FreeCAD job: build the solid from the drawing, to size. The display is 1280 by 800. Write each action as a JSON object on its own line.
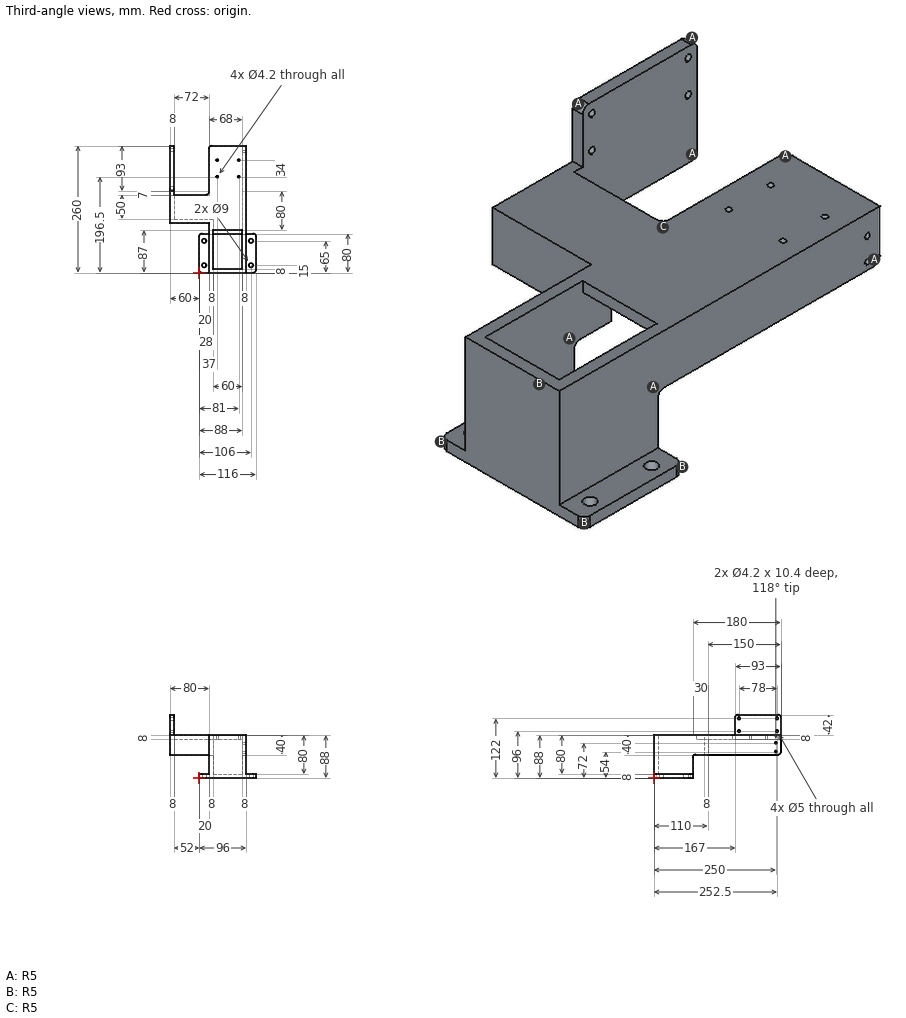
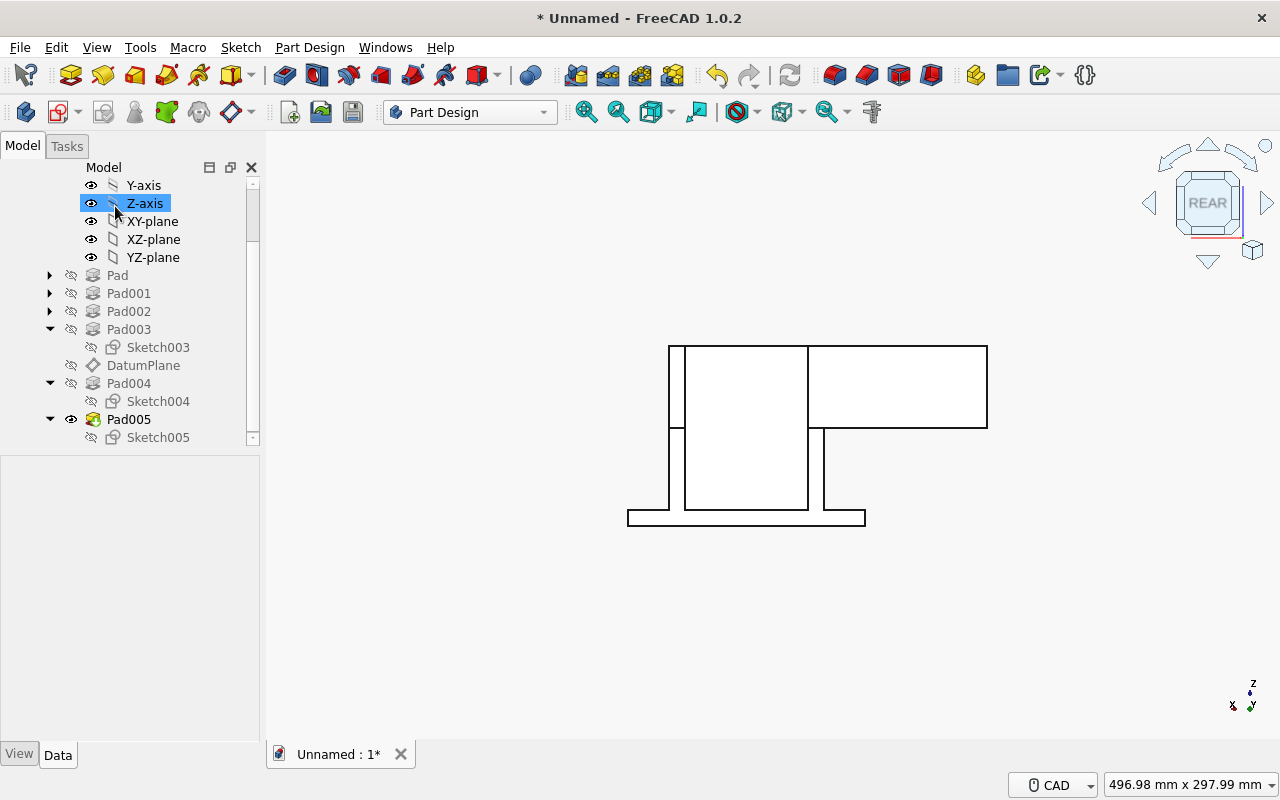
{"action": "left_click", "coordinate": [588, 112]}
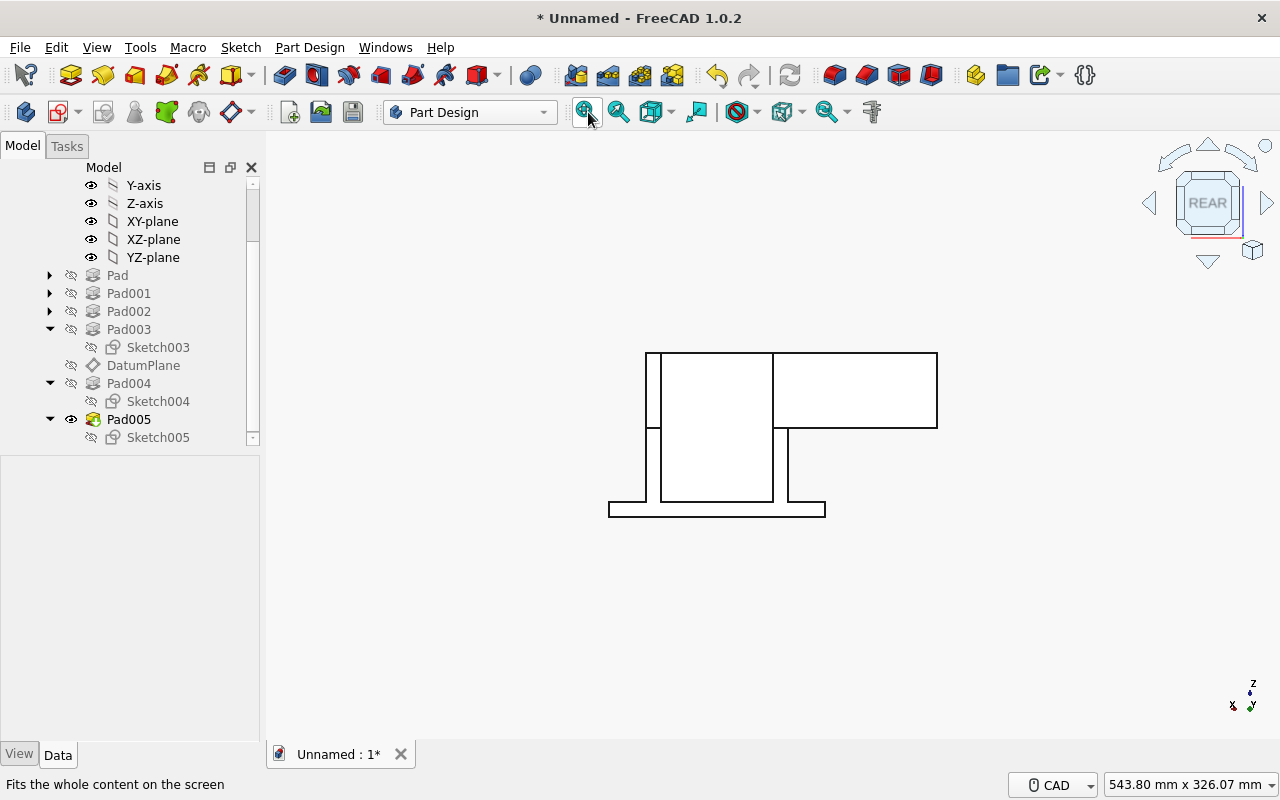
{"action": "left_click", "coordinate": [832, 389]}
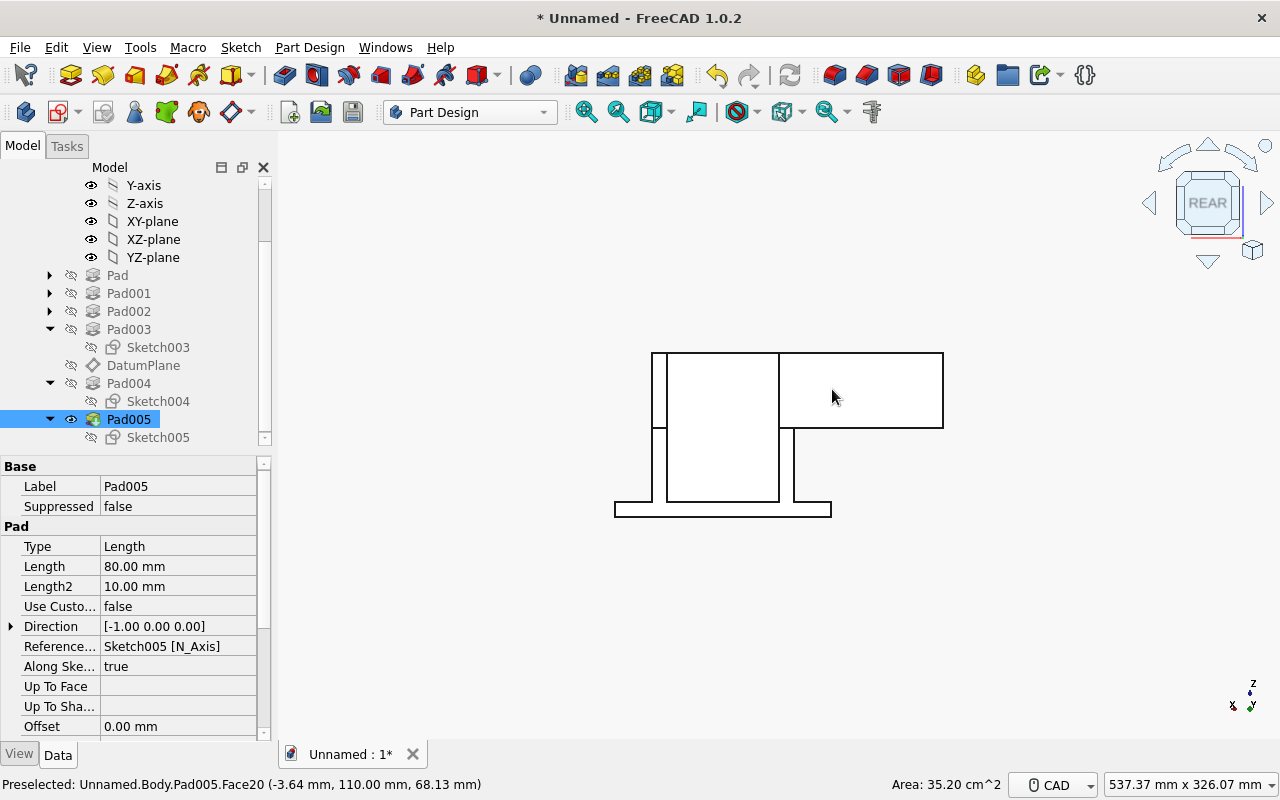
{"action": "left_click", "coordinate": [58, 112]}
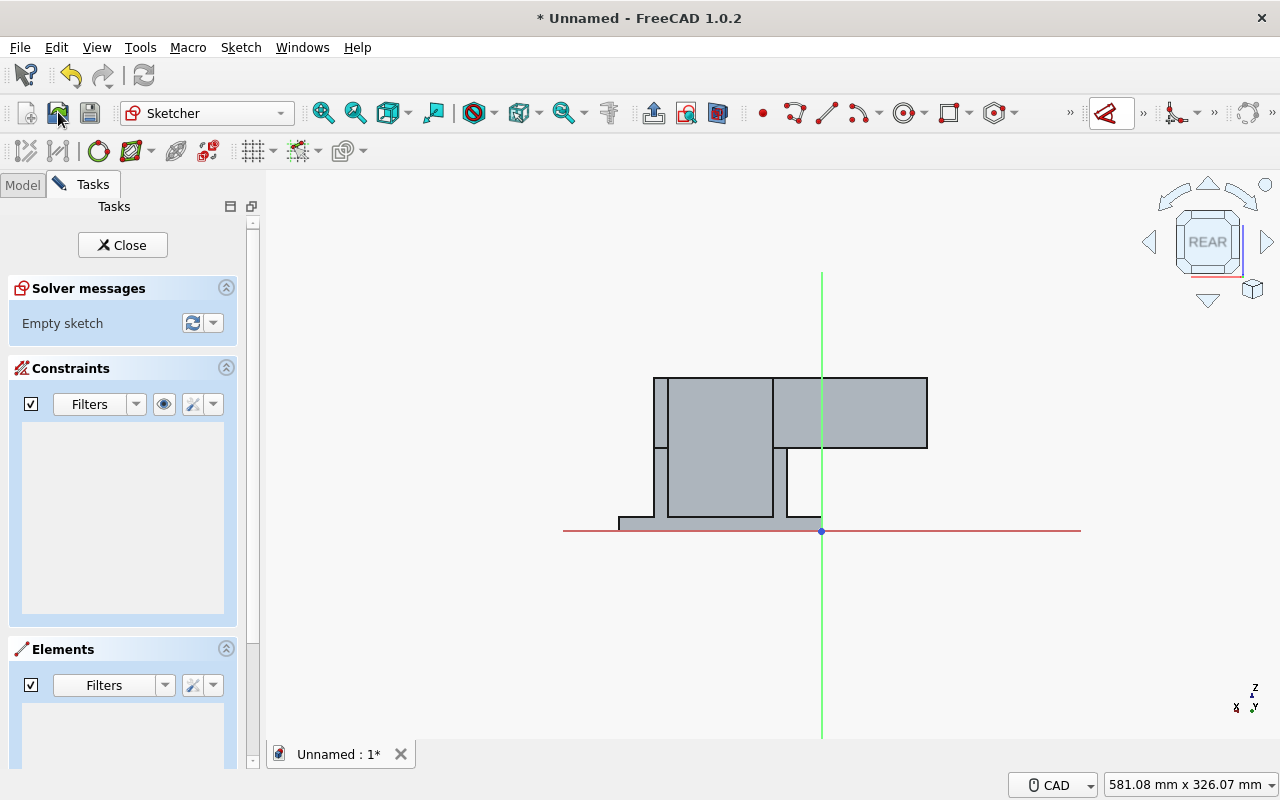
{"action": "scroll", "coordinate": [1013, 455], "scroll_direction": "up", "scroll_amount": 4}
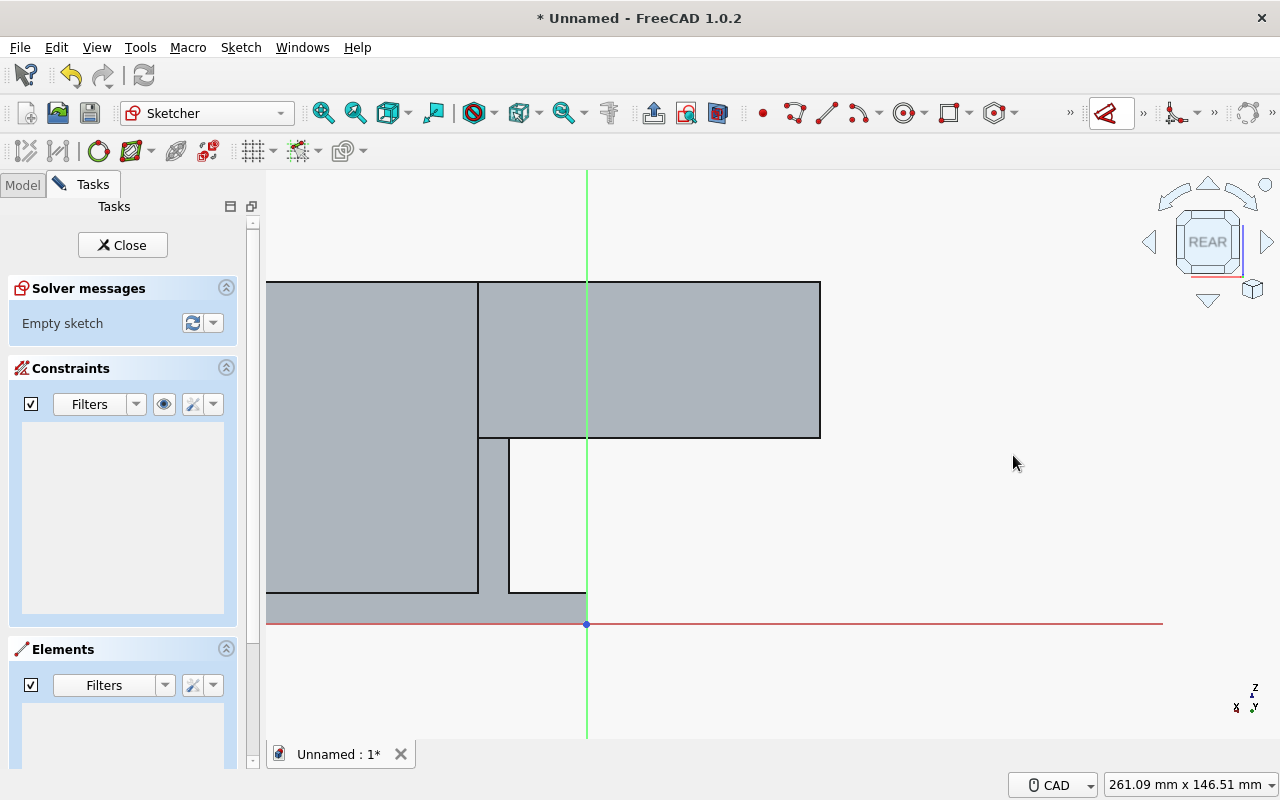
{"action": "left_click", "coordinate": [950, 114]}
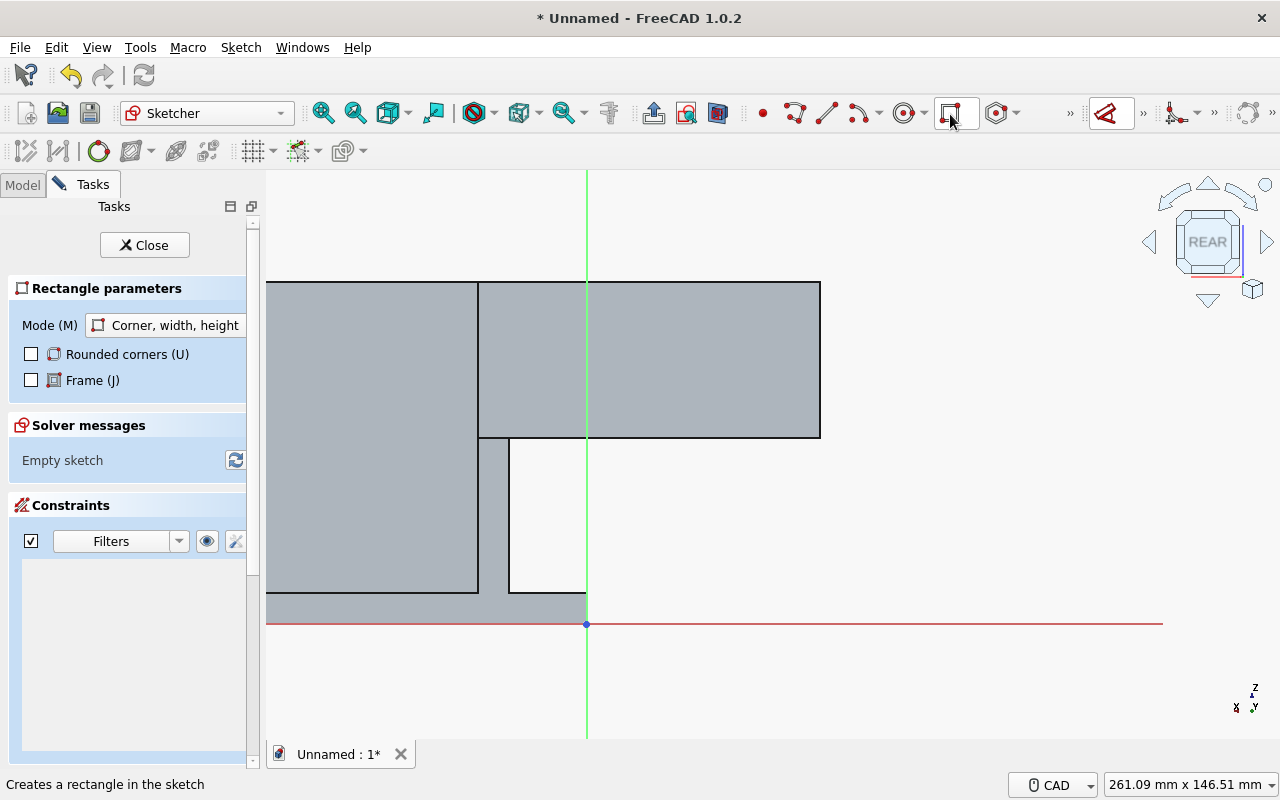
{"action": "left_click", "coordinate": [789, 282]}
{"action": "left_click", "coordinate": [820, 438]}
{"action": "key", "text": "Escape"}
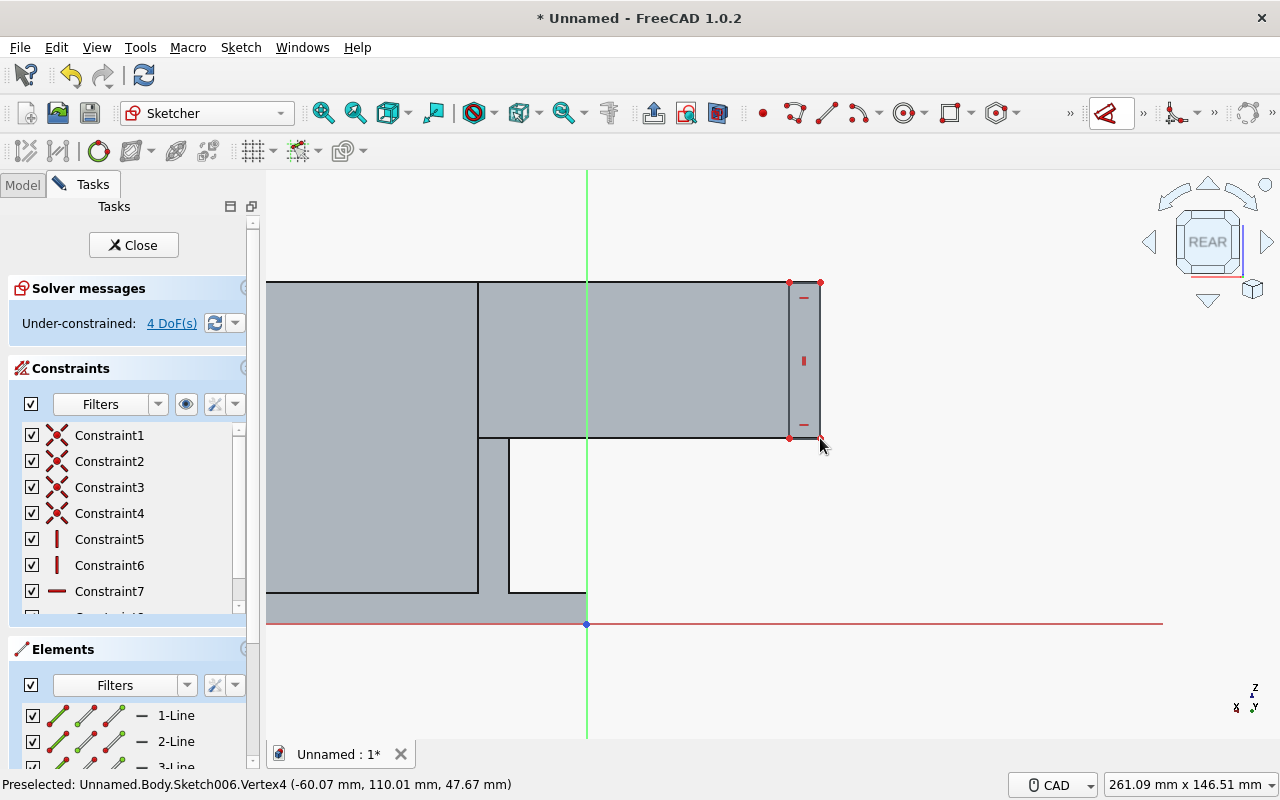
{"action": "scroll", "coordinate": [798, 439], "scroll_direction": "up", "scroll_amount": 2}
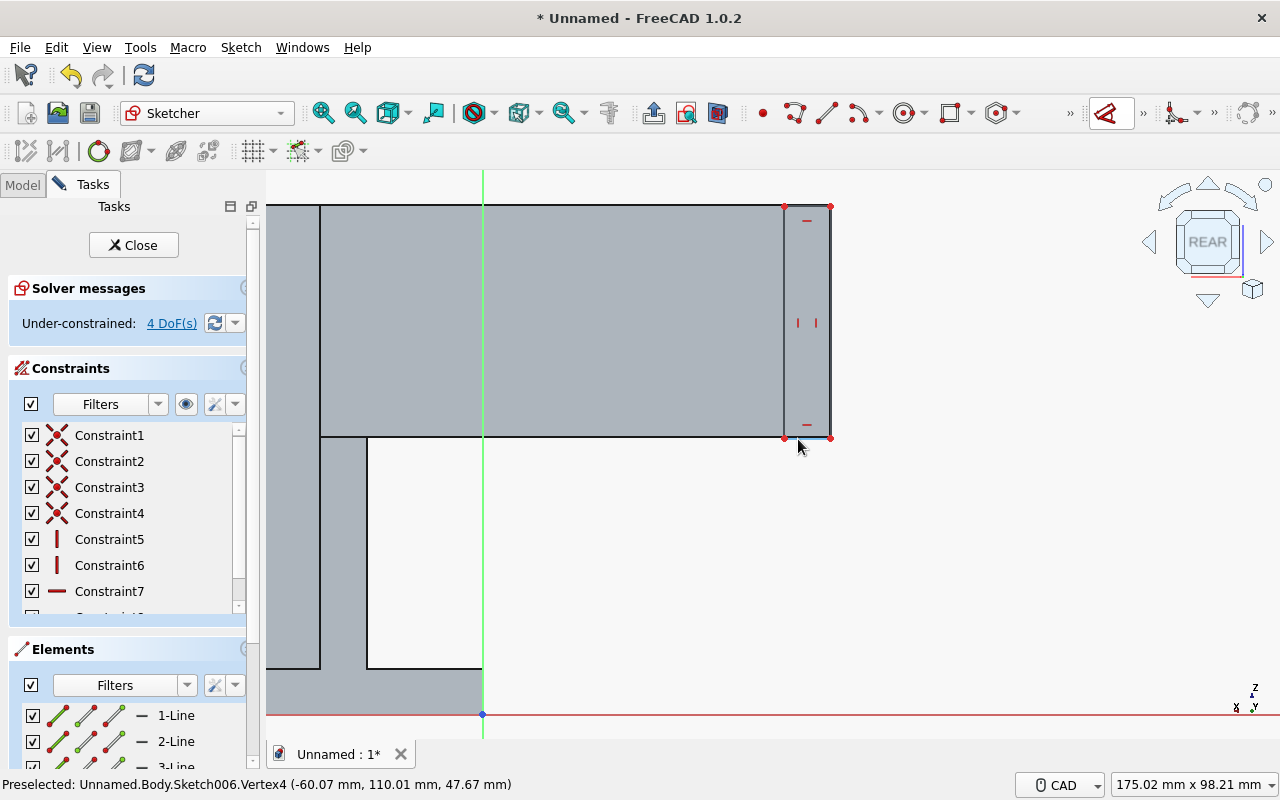
{"action": "left_click", "coordinate": [798, 439]}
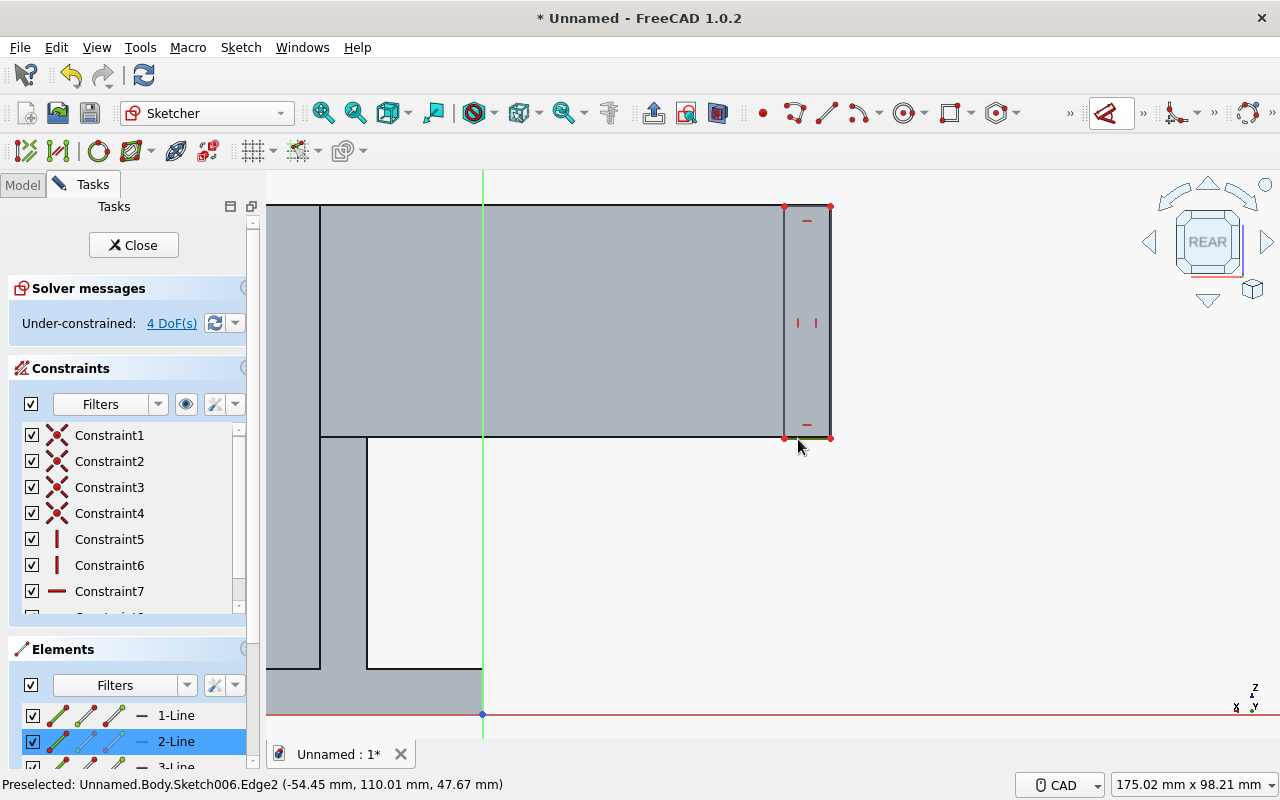
{"action": "key", "text": "l"}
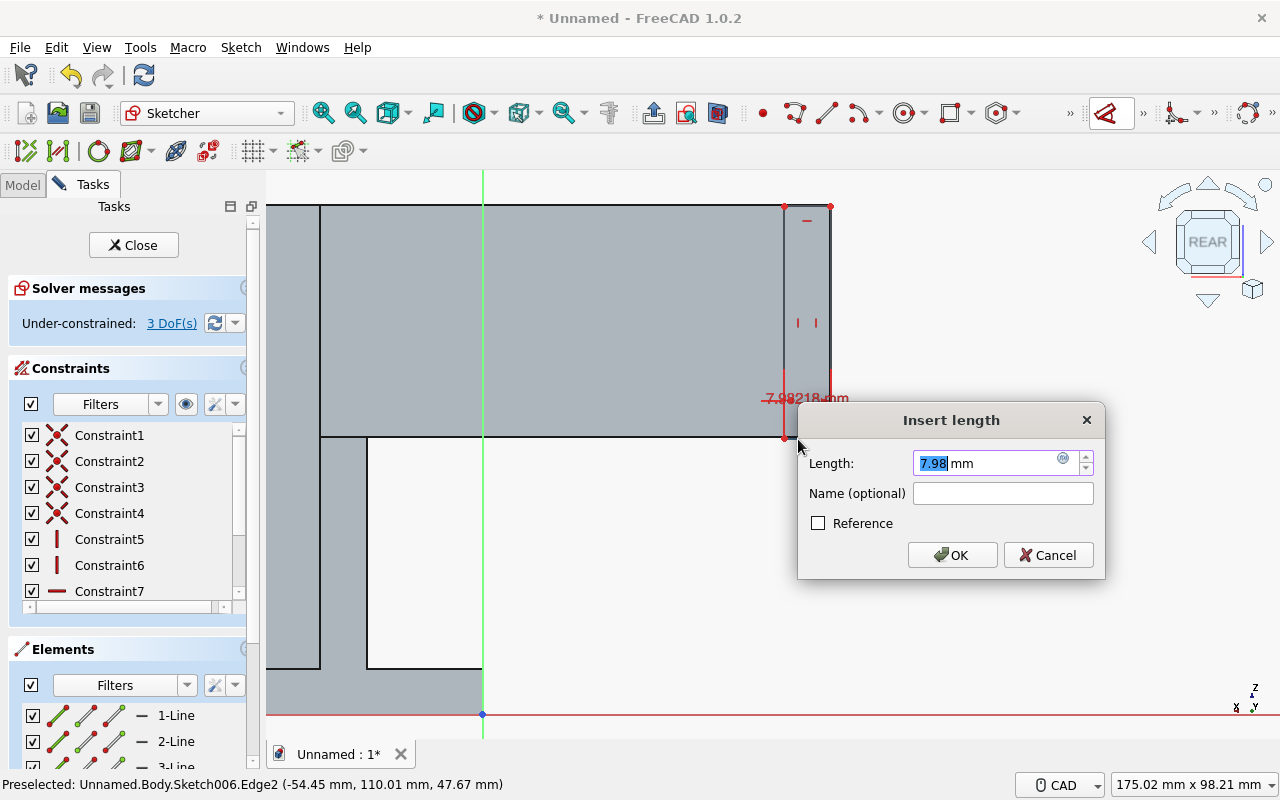
{"action": "type", "text": "8"}
{"action": "key", "text": "Return"}